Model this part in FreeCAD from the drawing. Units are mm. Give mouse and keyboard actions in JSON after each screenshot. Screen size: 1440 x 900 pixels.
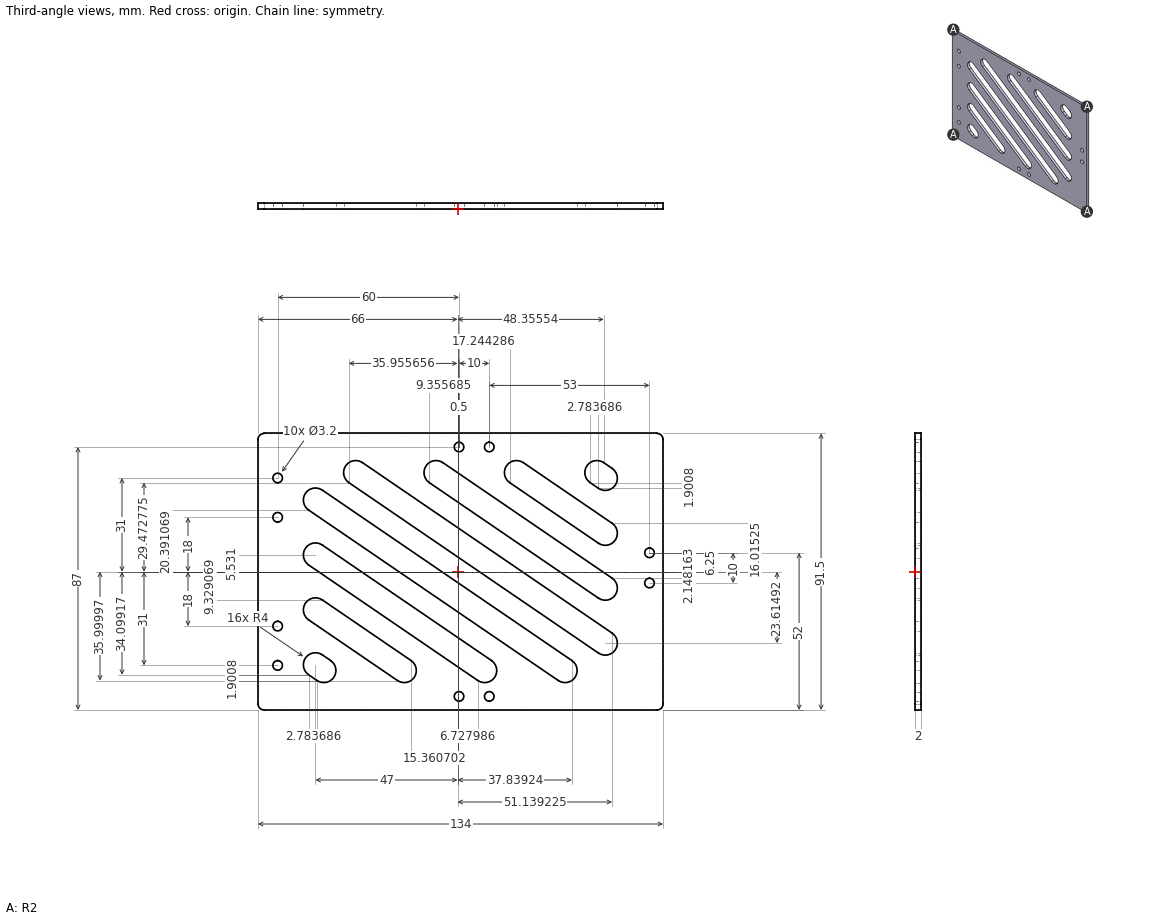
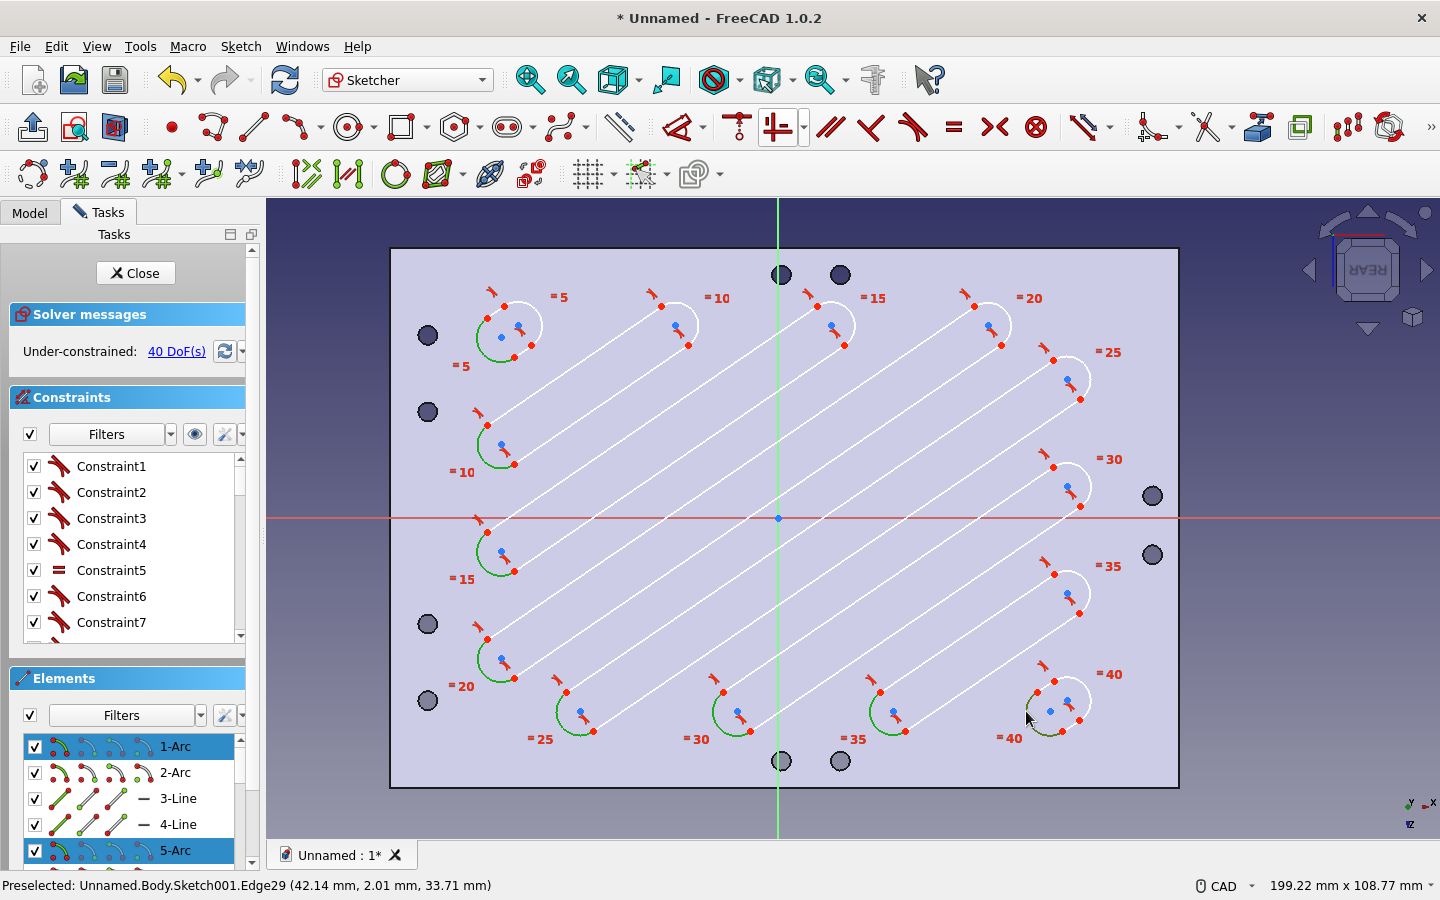
{"action": "left_click", "coordinate": [954, 128]}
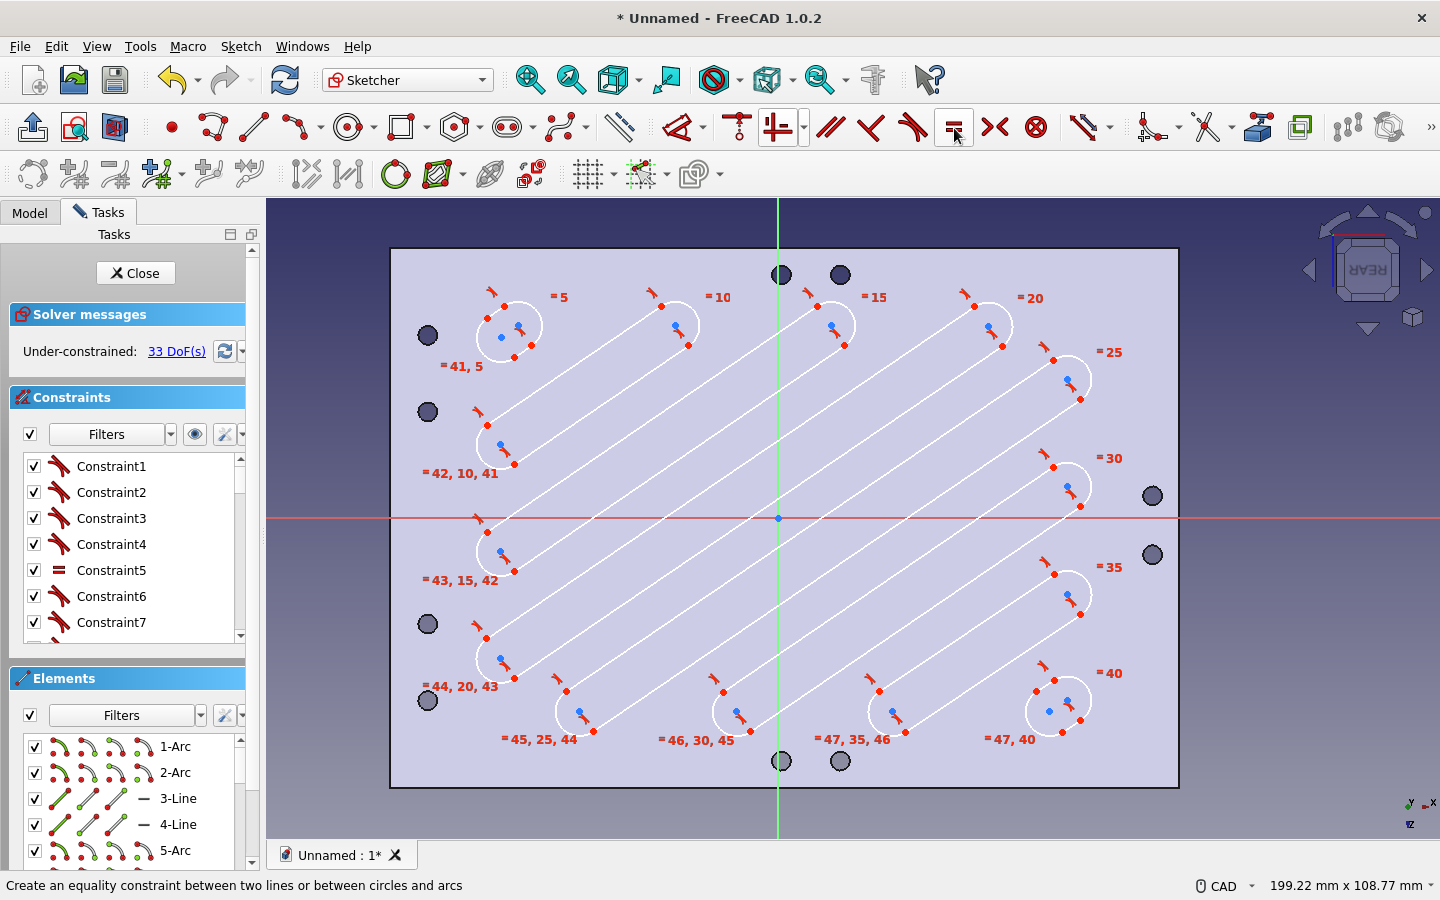
{"action": "left_click", "coordinate": [676, 128]}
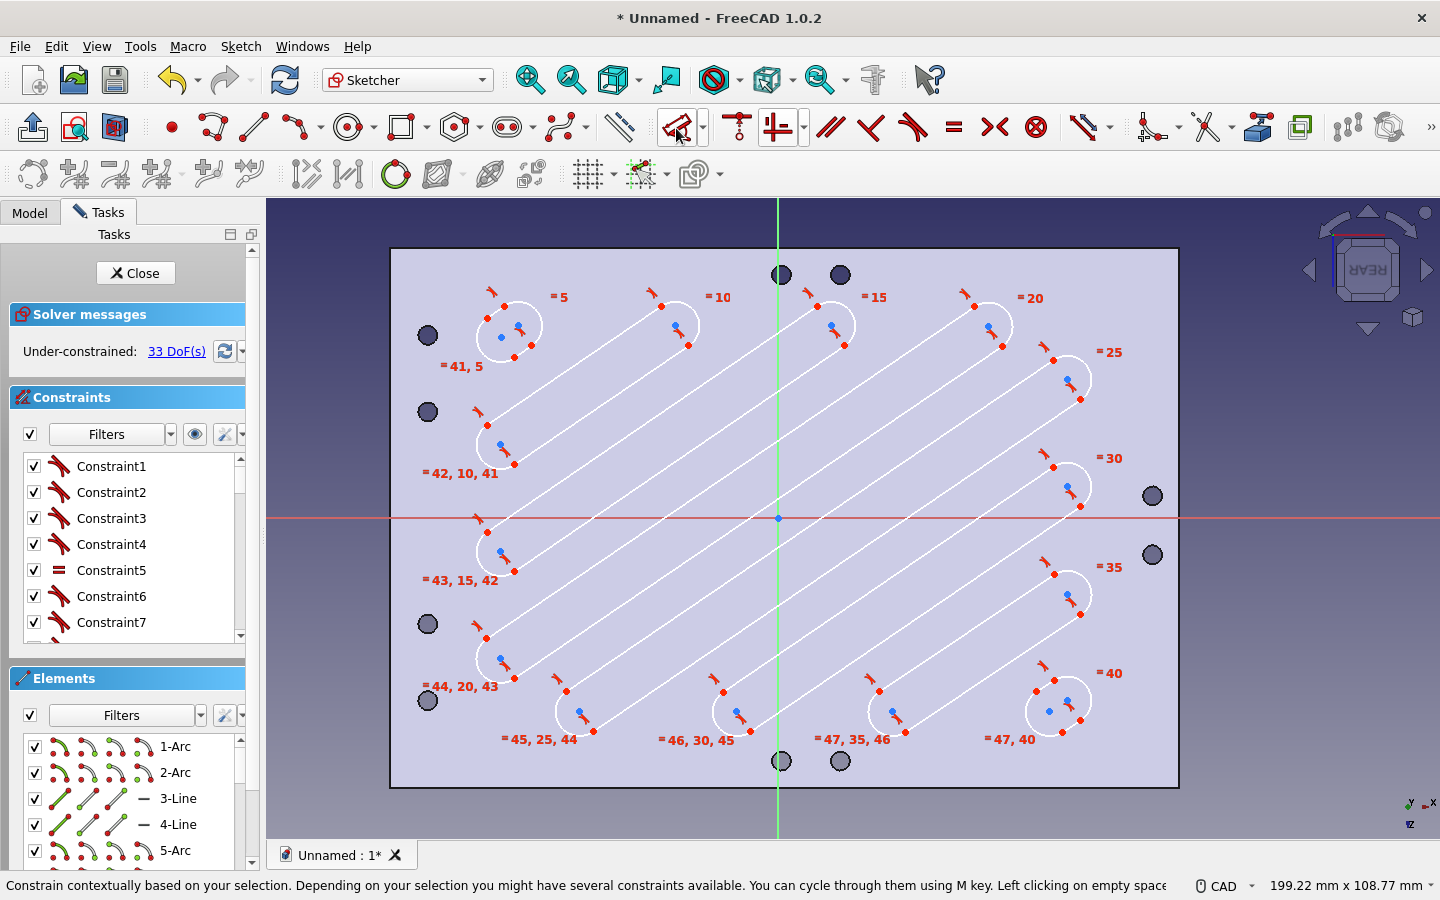
{"action": "scroll", "coordinate": [477, 338], "scroll_direction": "up", "scroll_amount": 3}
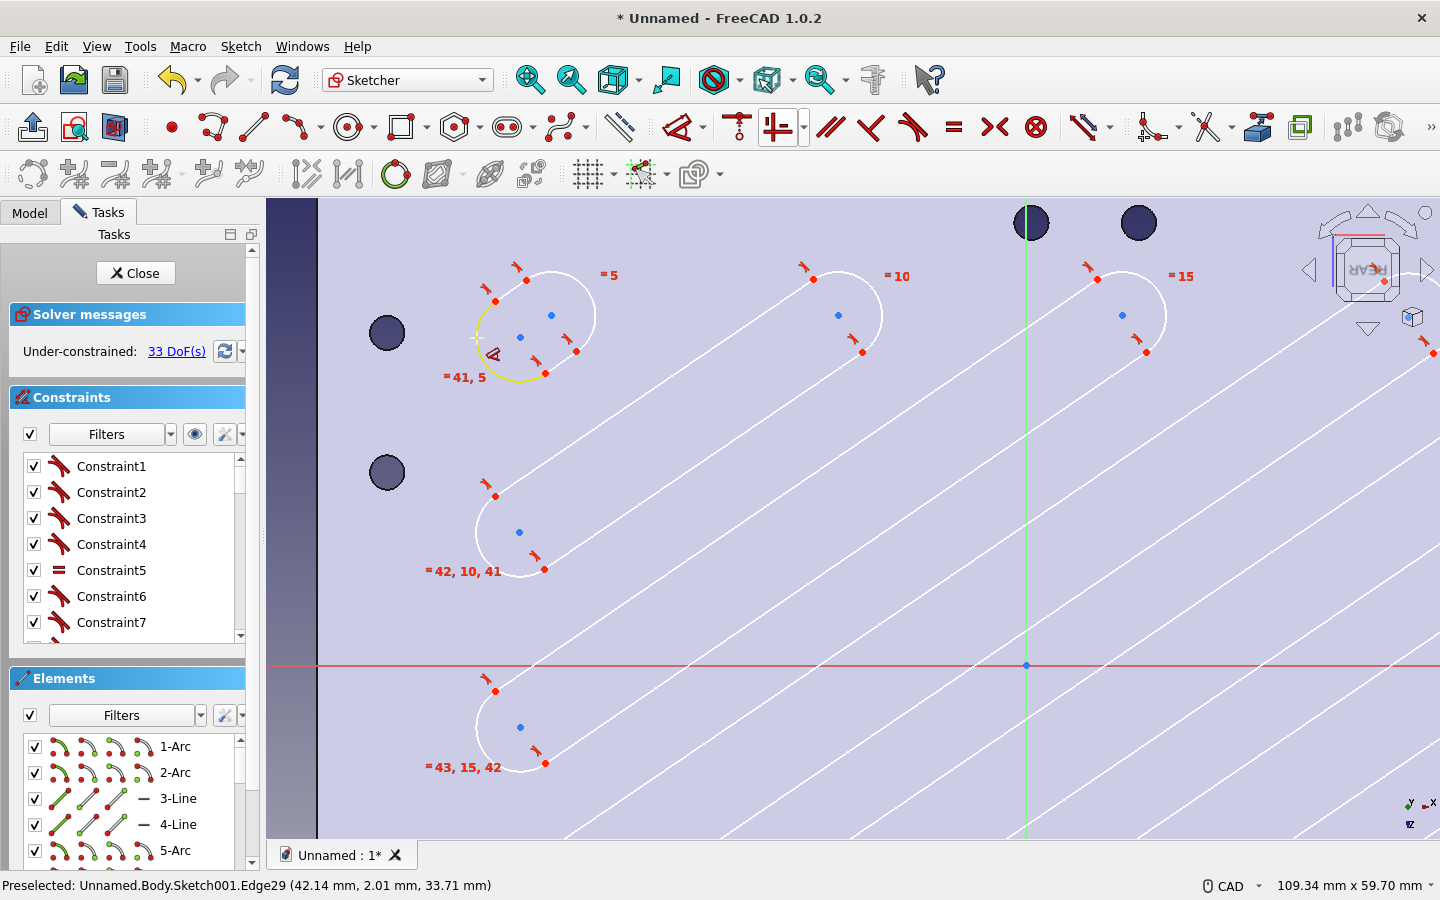
{"action": "left_click", "coordinate": [477, 337]}
{"action": "left_click", "coordinate": [445, 336]}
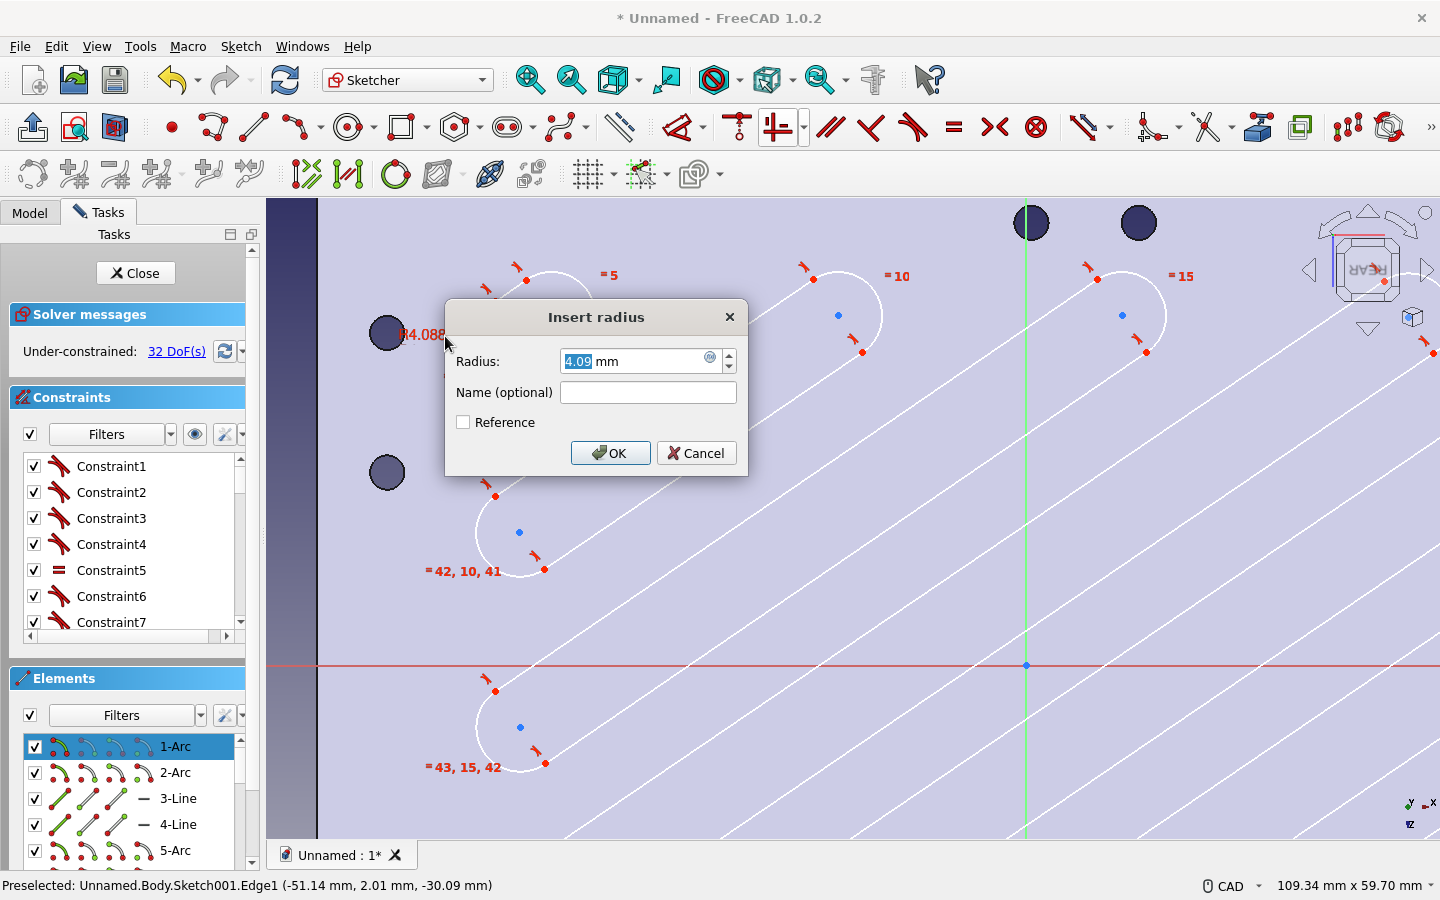
{"action": "type", "text": "4"}
{"action": "key", "text": "Return"}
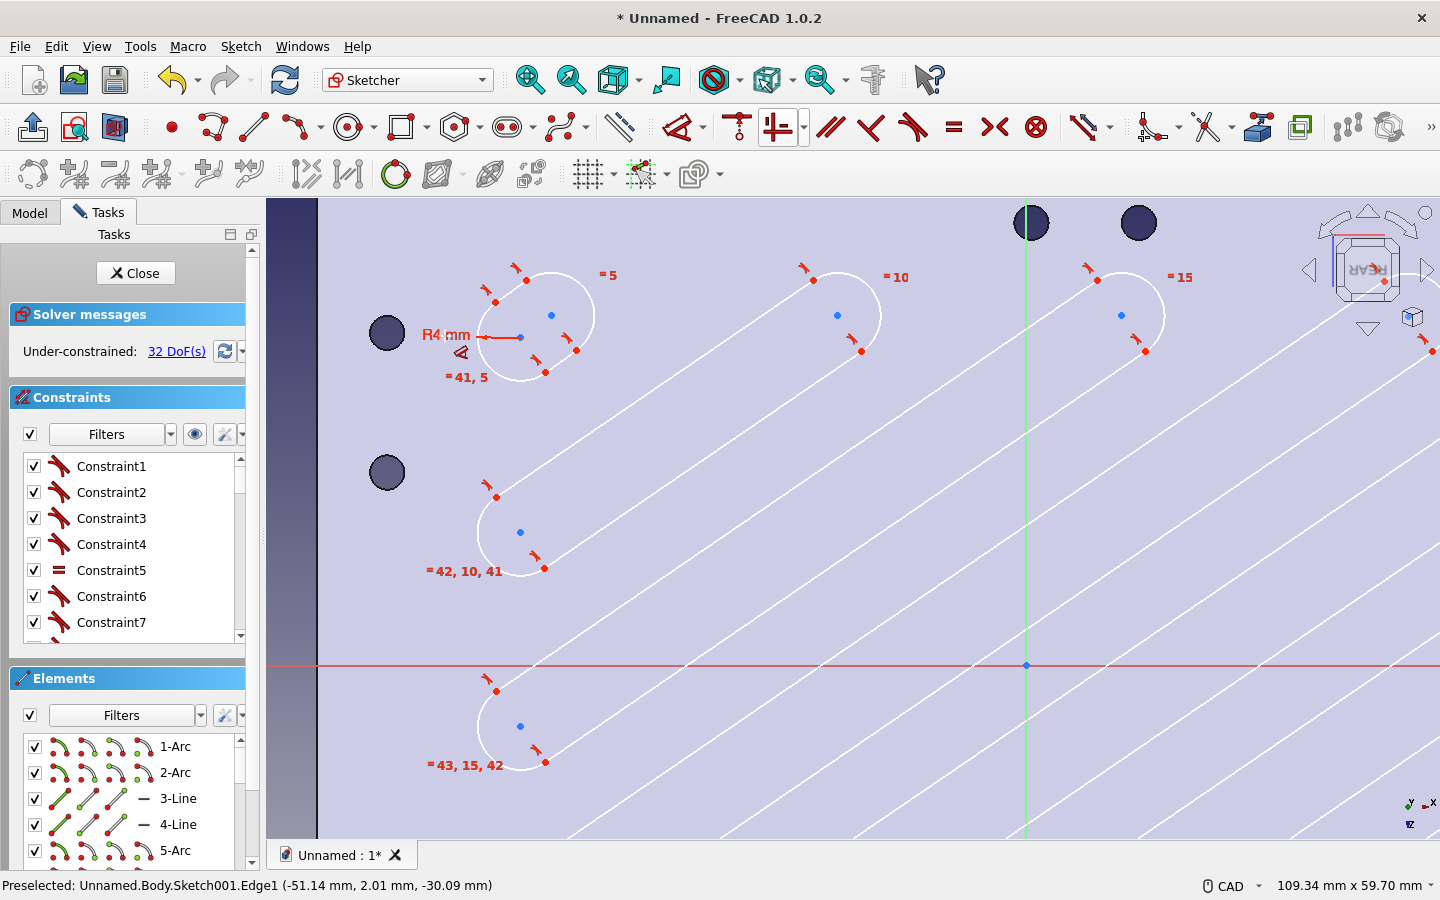
{"action": "left_click", "coordinate": [521, 338]}
{"action": "left_click", "coordinate": [657, 304]}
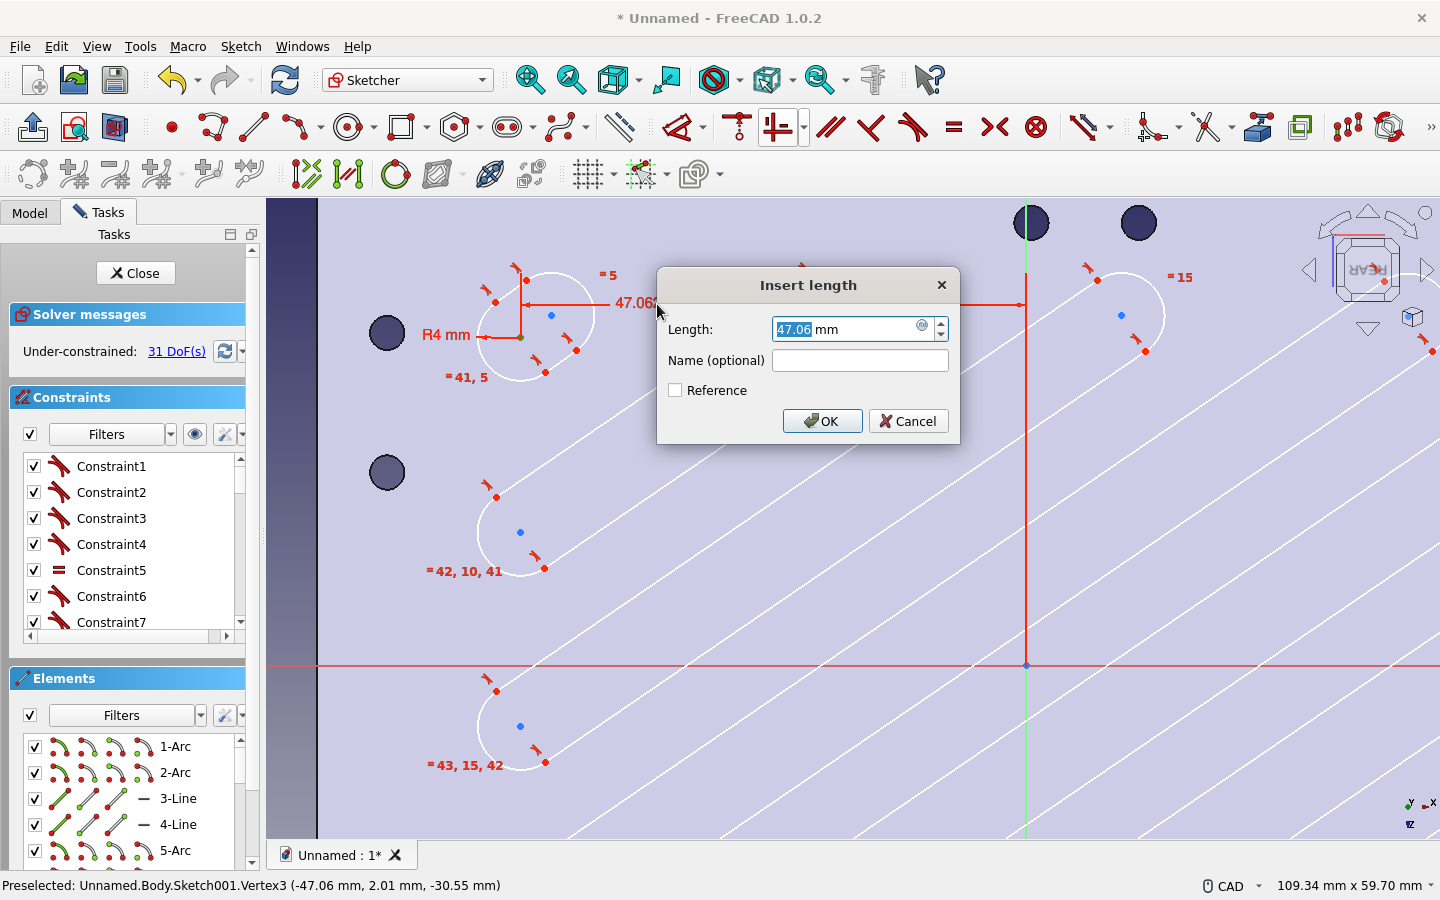
{"action": "type", "text": "47"}
{"action": "key", "text": "Return"}